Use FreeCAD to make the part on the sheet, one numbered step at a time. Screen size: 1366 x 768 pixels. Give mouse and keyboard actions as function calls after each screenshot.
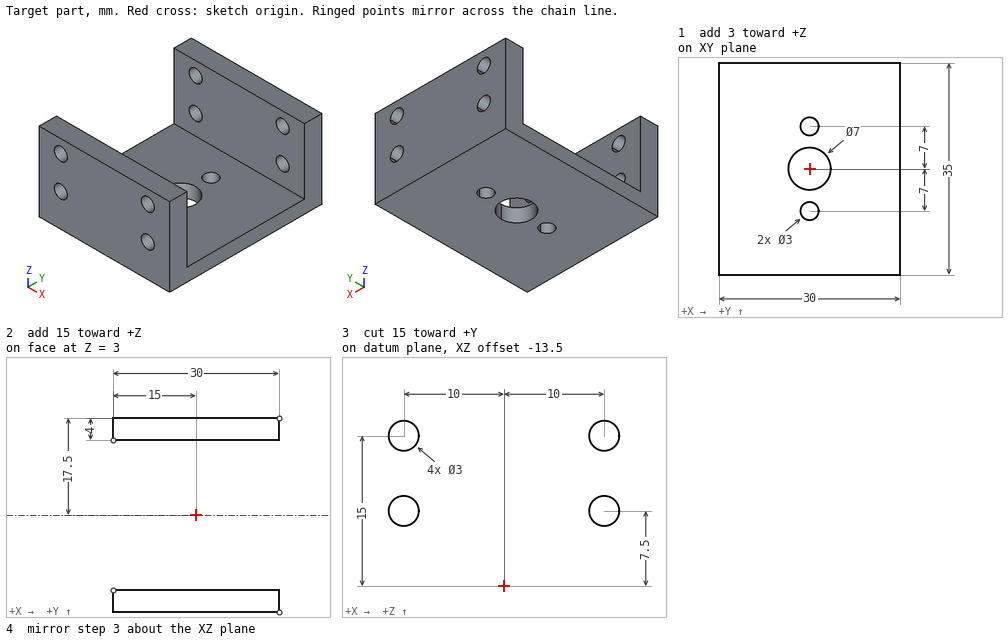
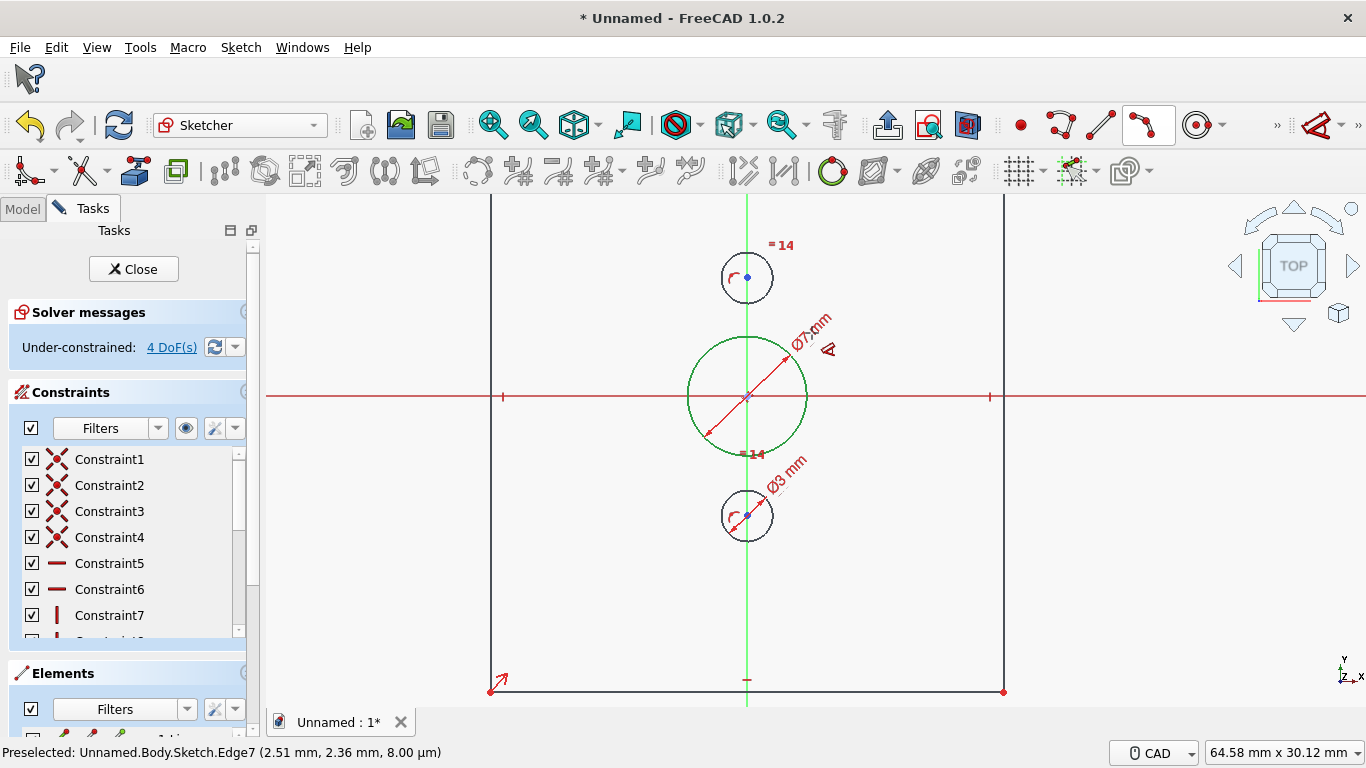
click(747, 516)
click(781, 414)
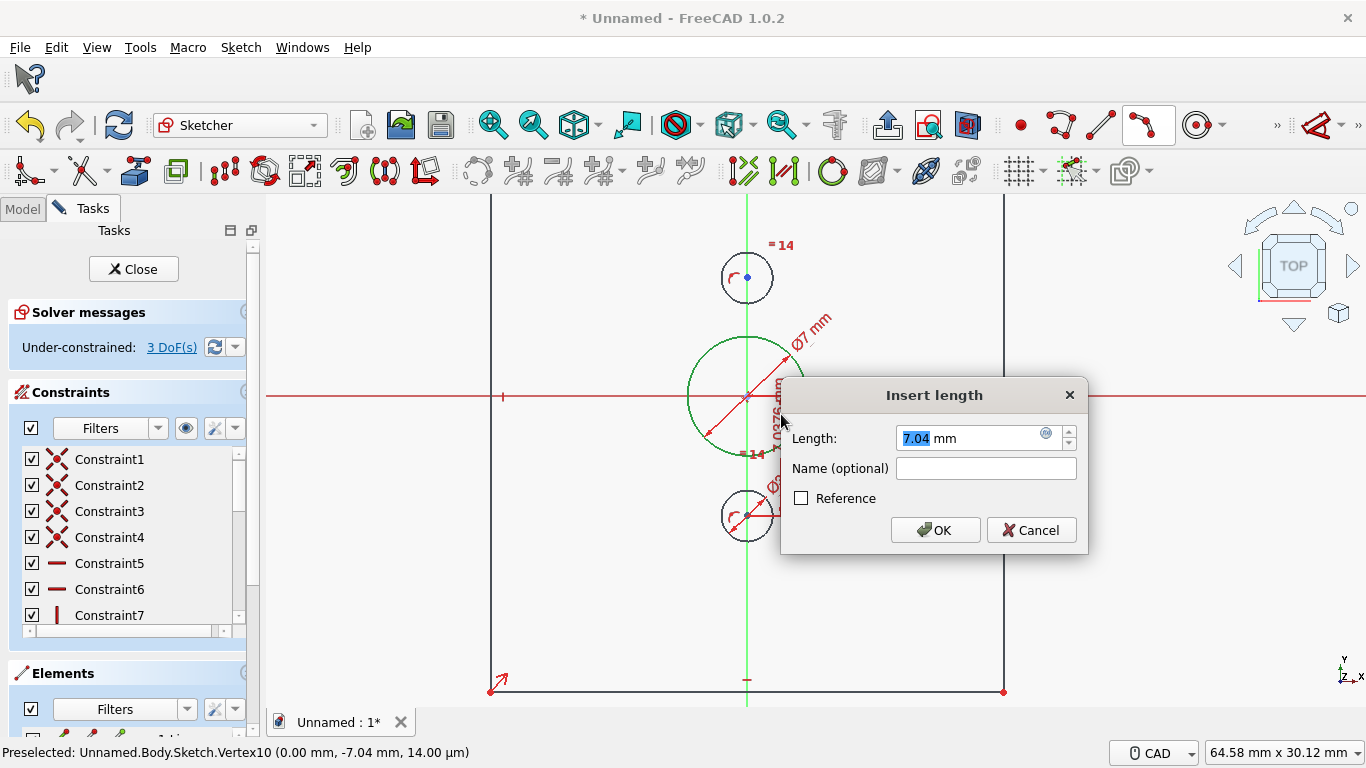
text(7)
key(Return)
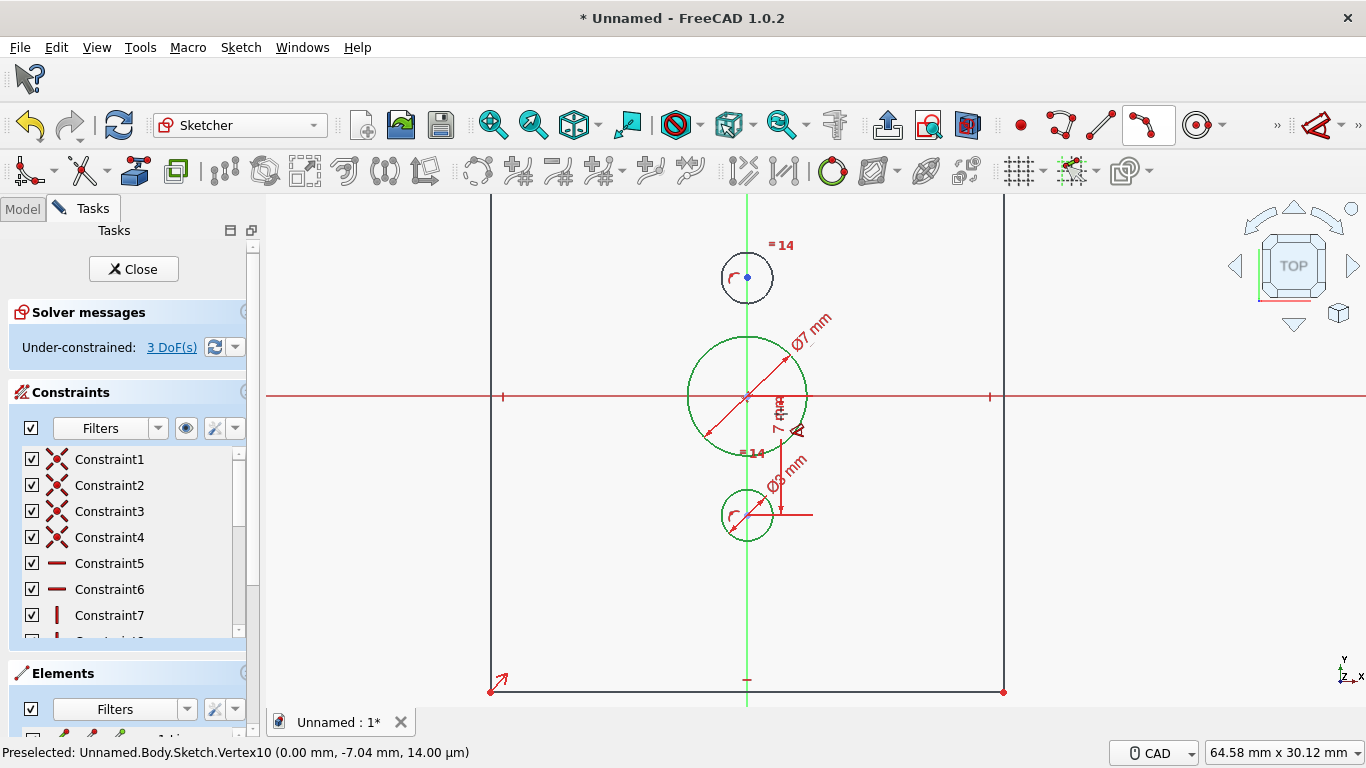
click(747, 278)
click(781, 310)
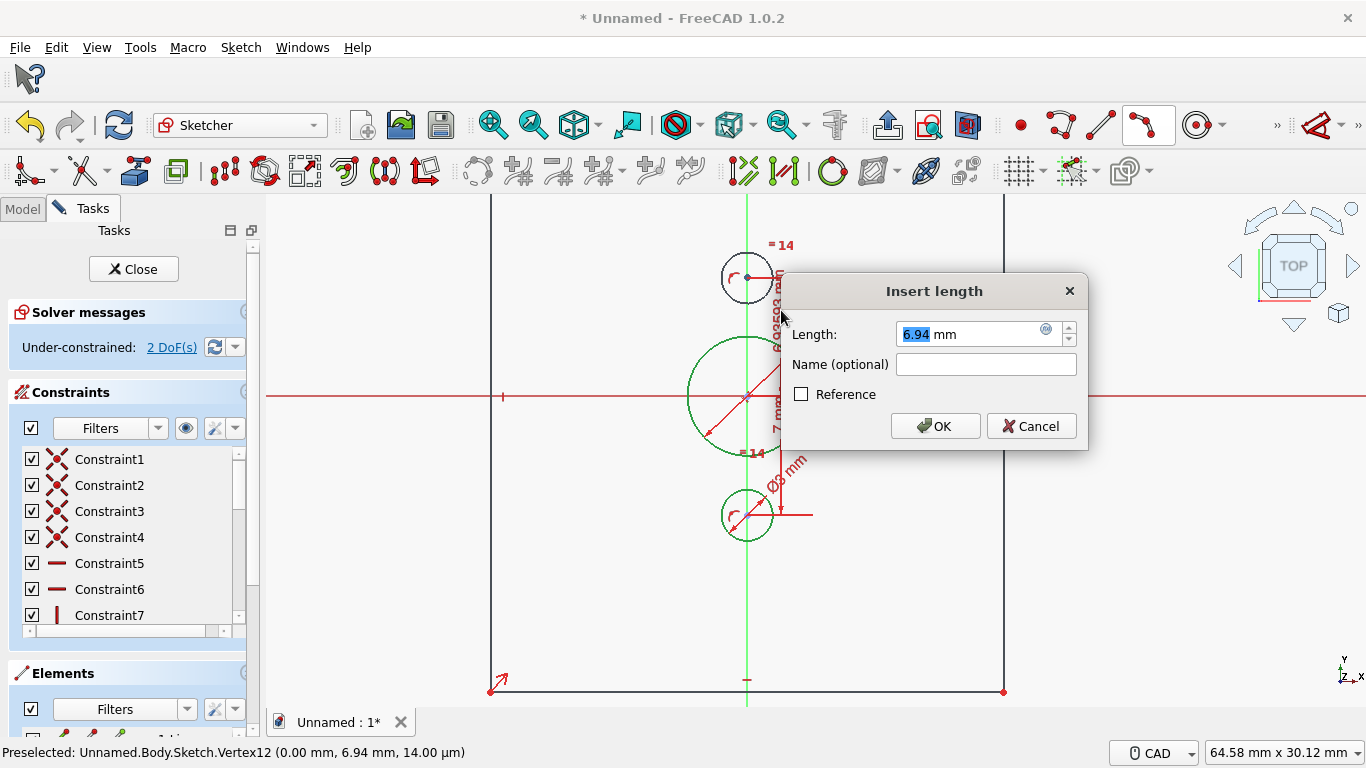
text(7)
key(Return)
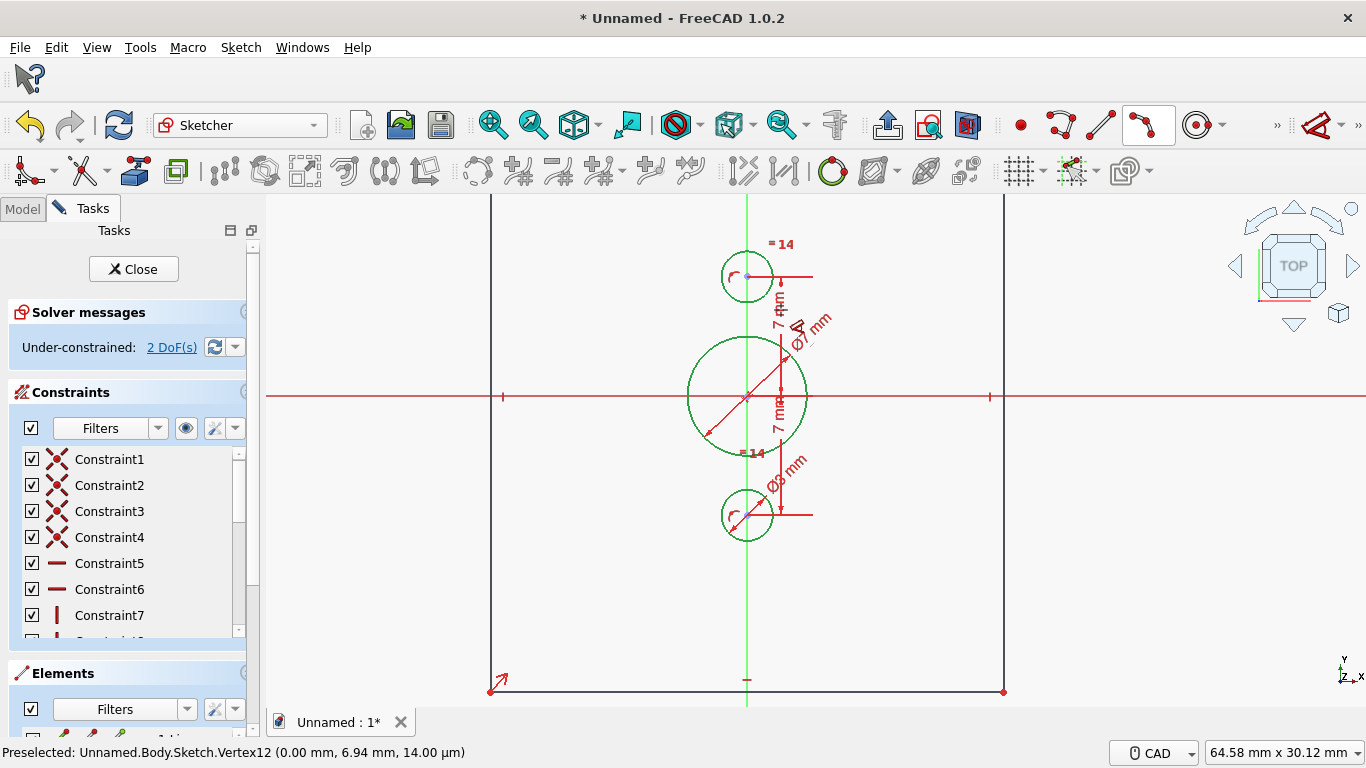
scroll(748, 517, down, 3)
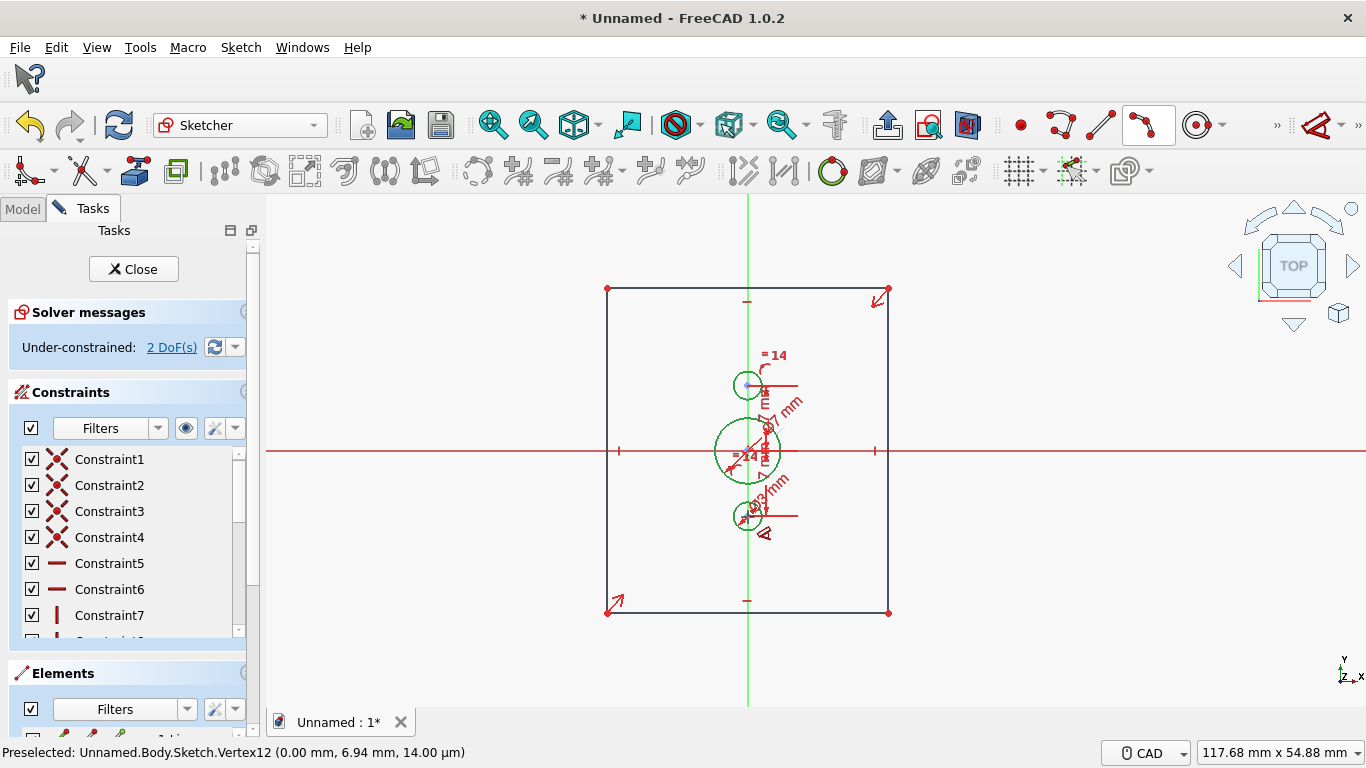
click(691, 613)
click(683, 647)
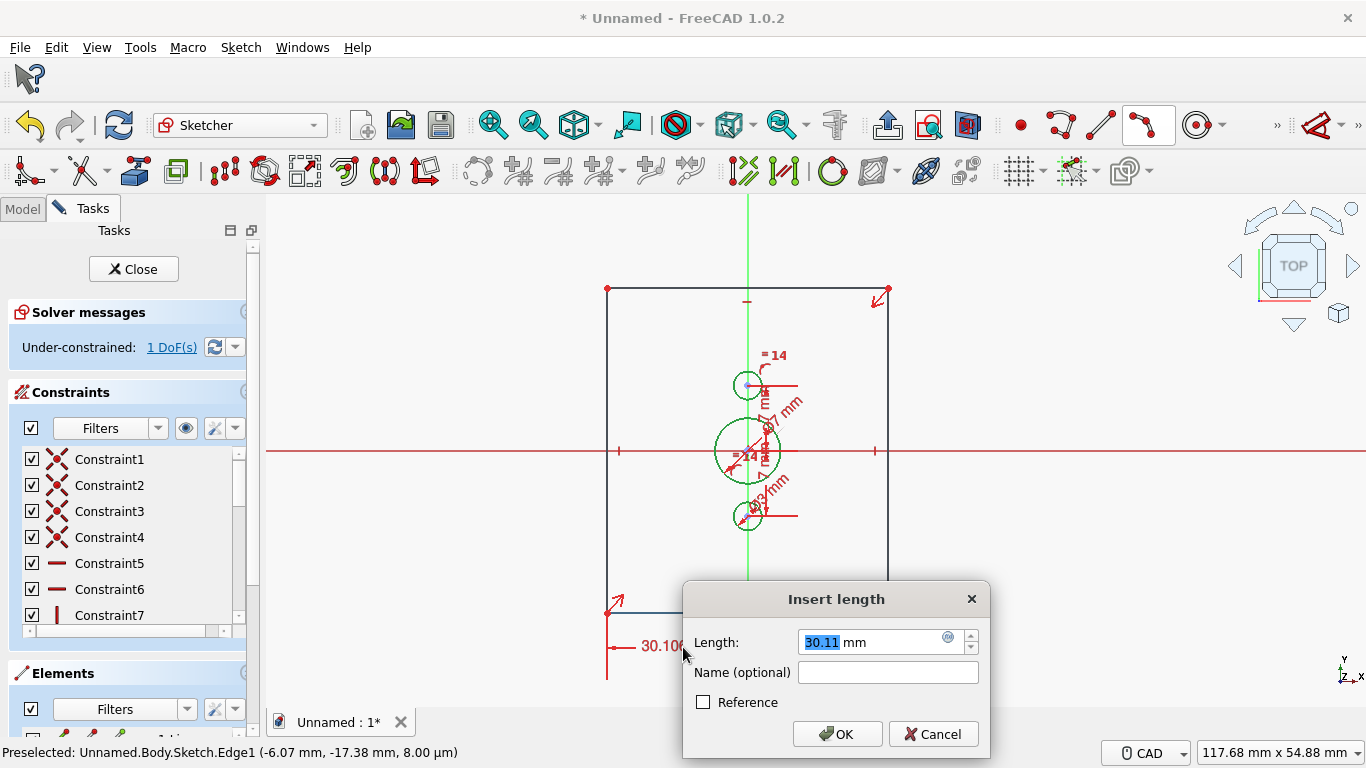
text(30)
key(Return)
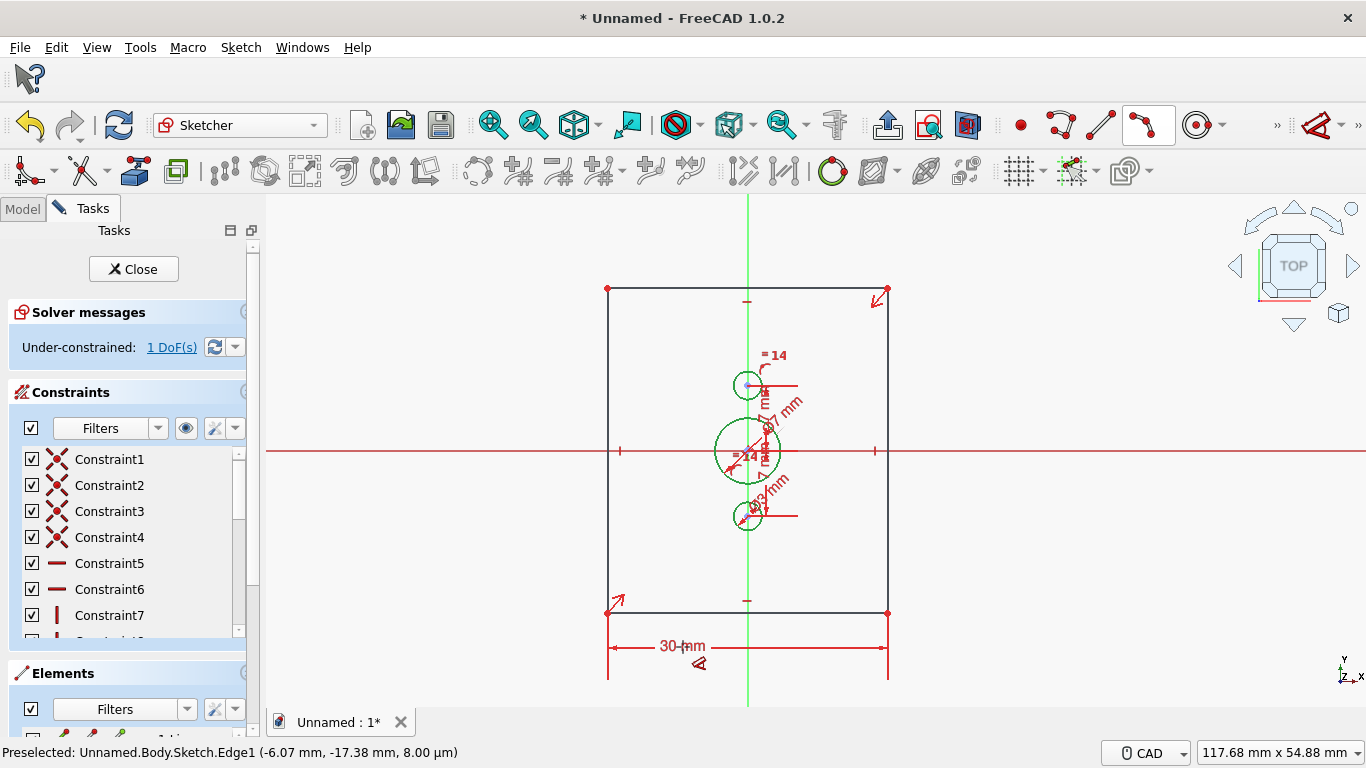
click(888, 516)
click(922, 376)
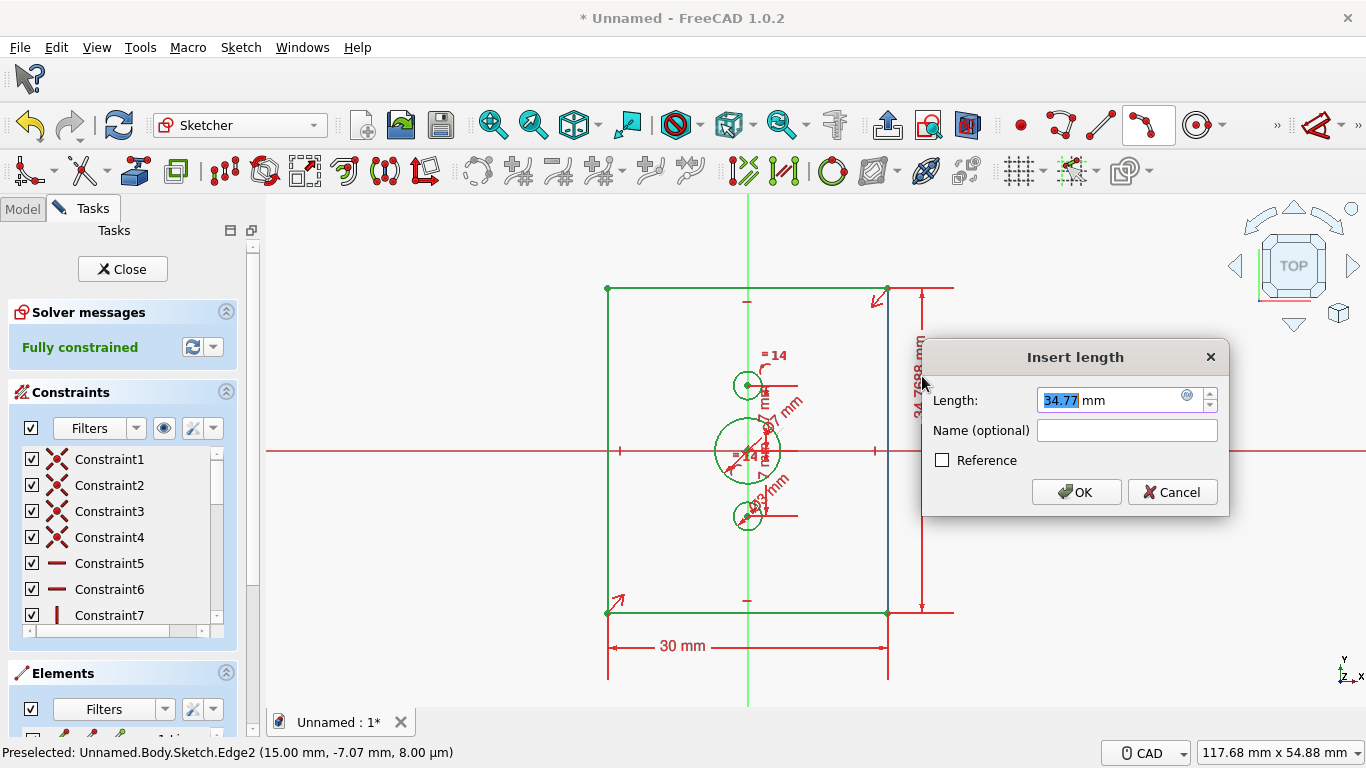
text(35)
key(Return)
key(Escape)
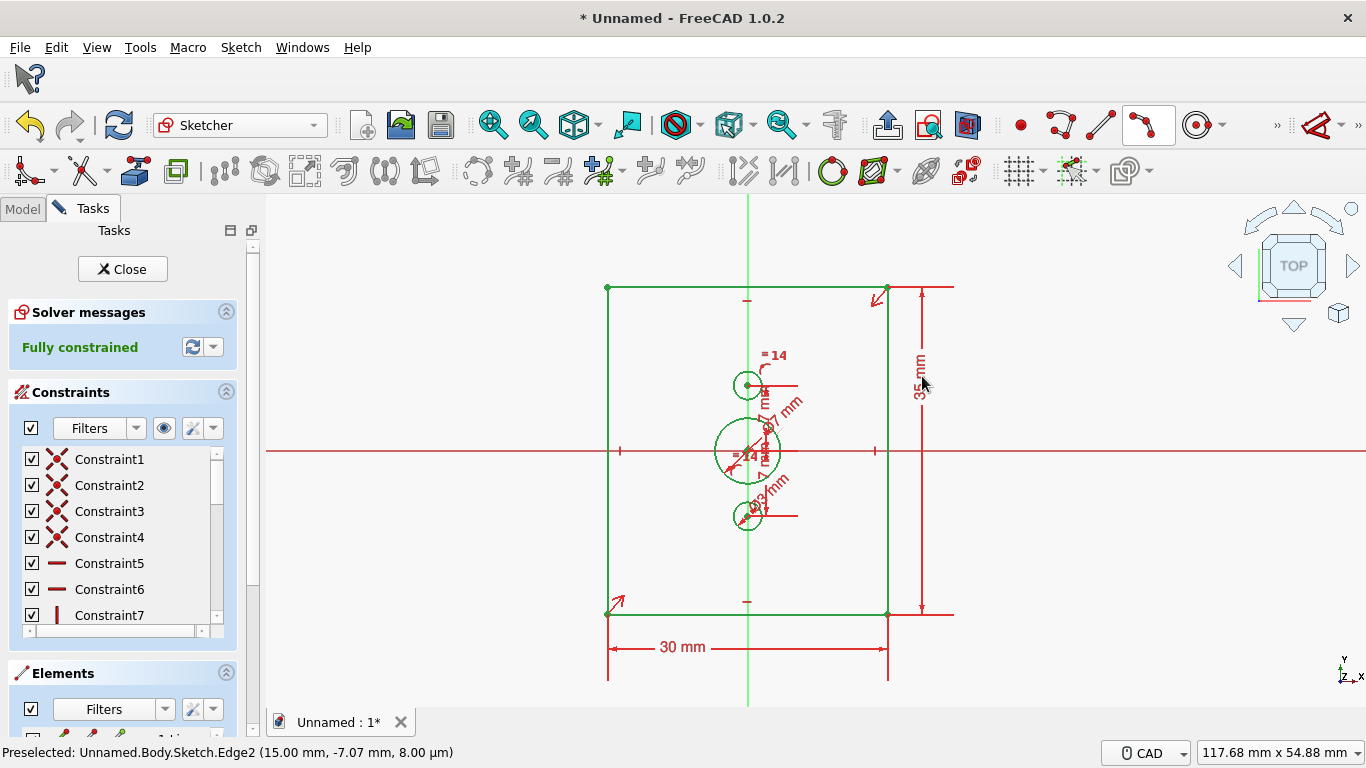
click(123, 269)